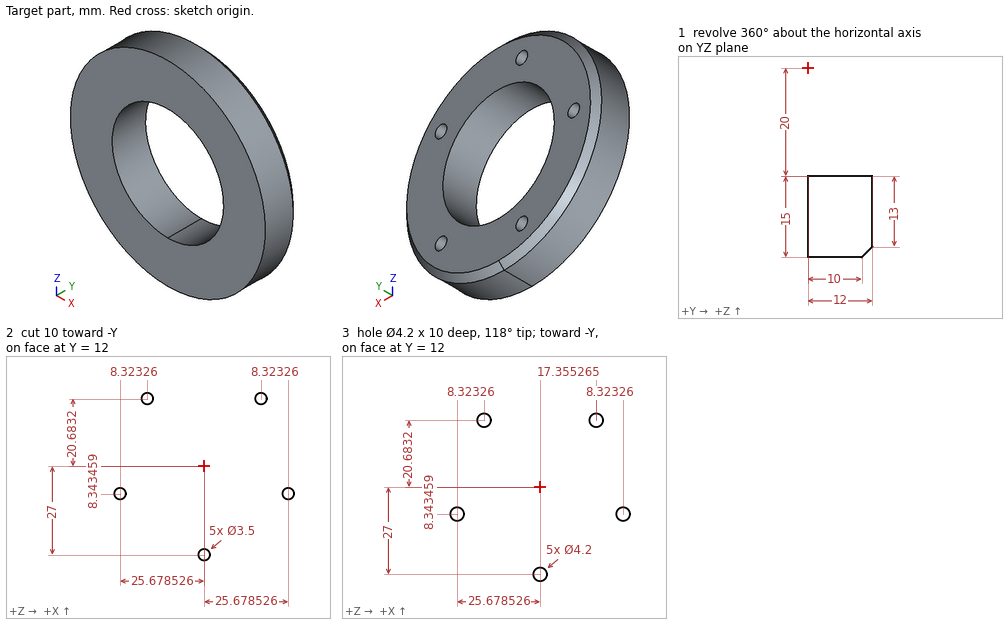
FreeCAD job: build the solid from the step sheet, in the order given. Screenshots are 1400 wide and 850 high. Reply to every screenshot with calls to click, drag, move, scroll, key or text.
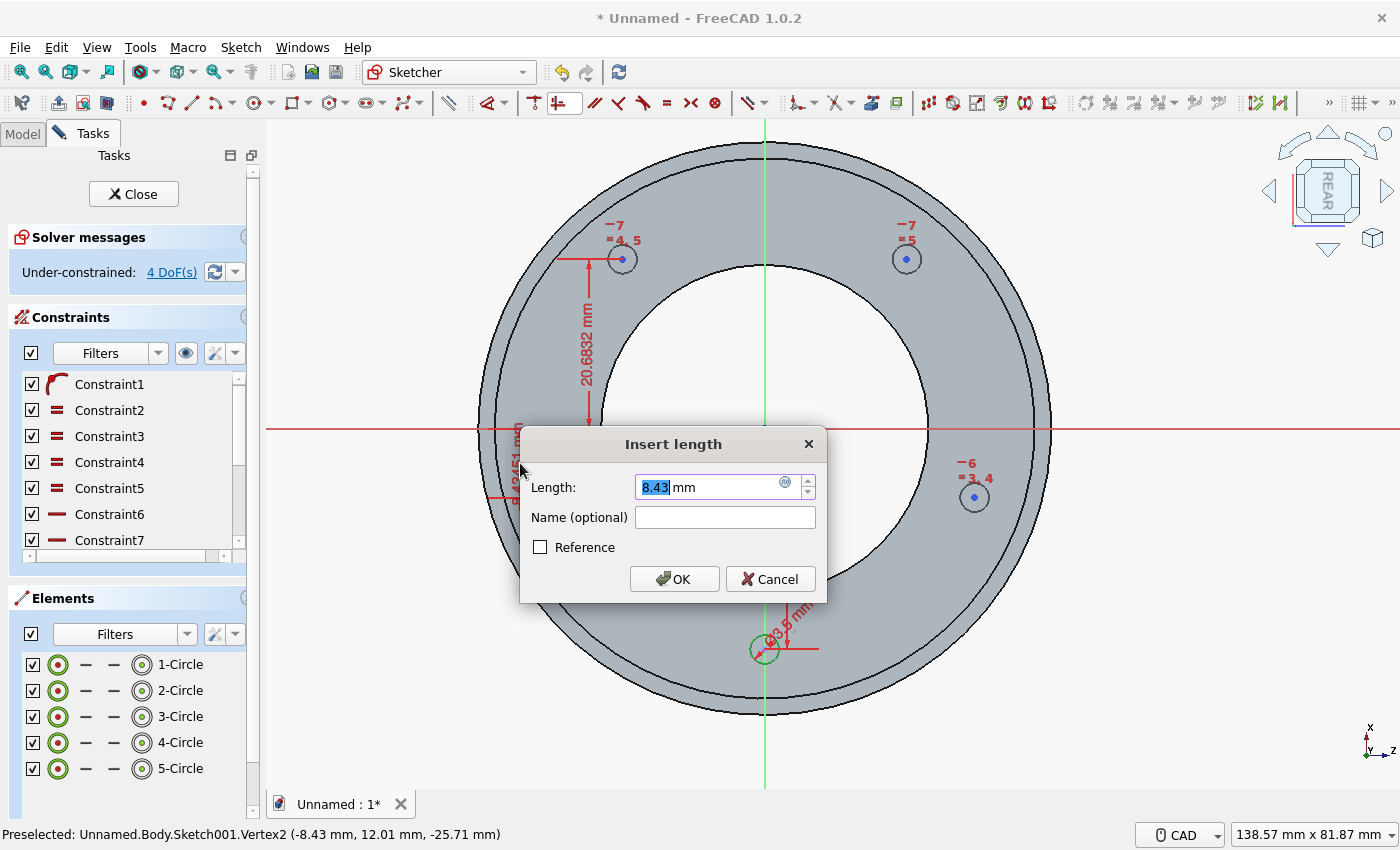
text(8.343459)
key(Return)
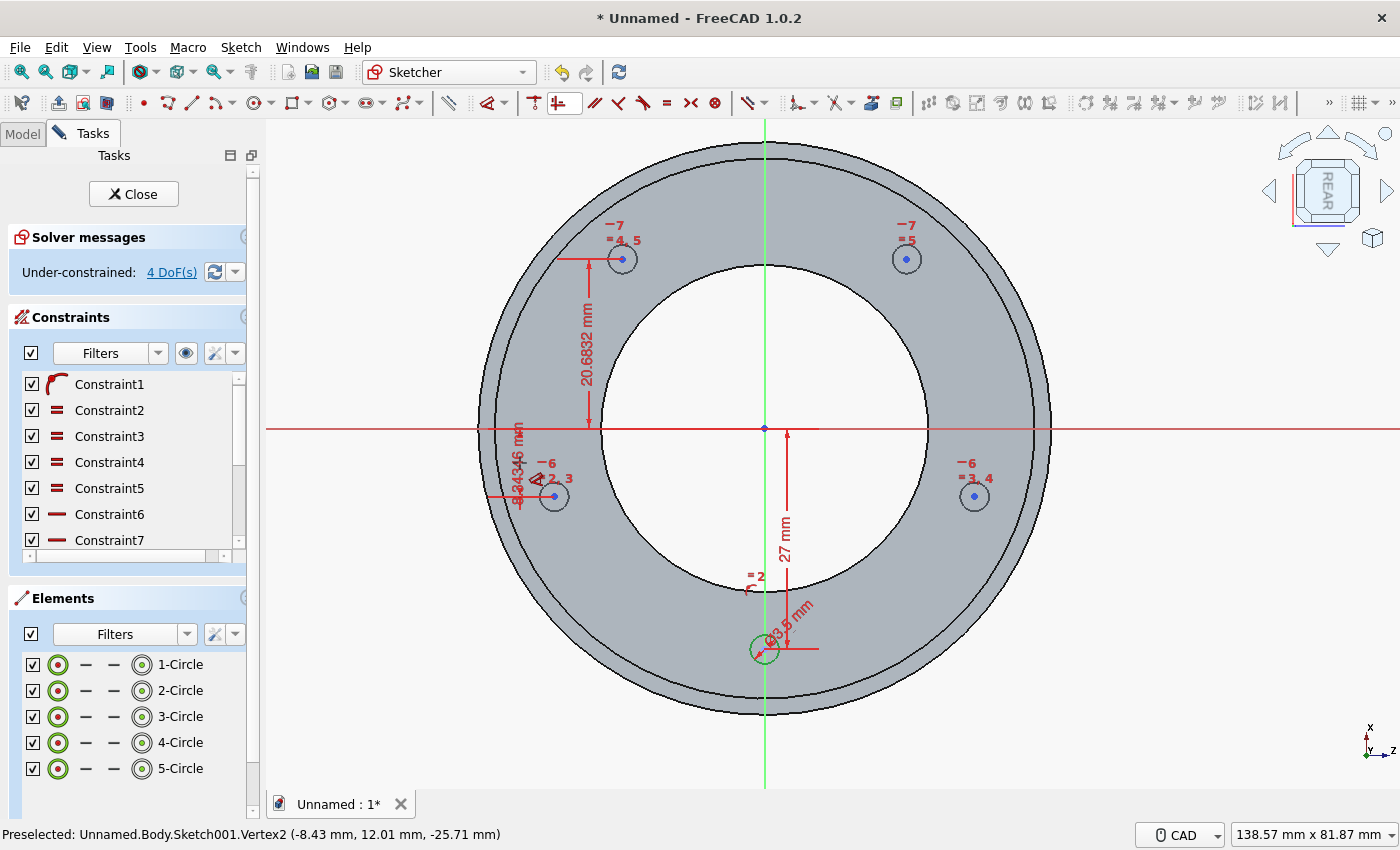
click(554, 497)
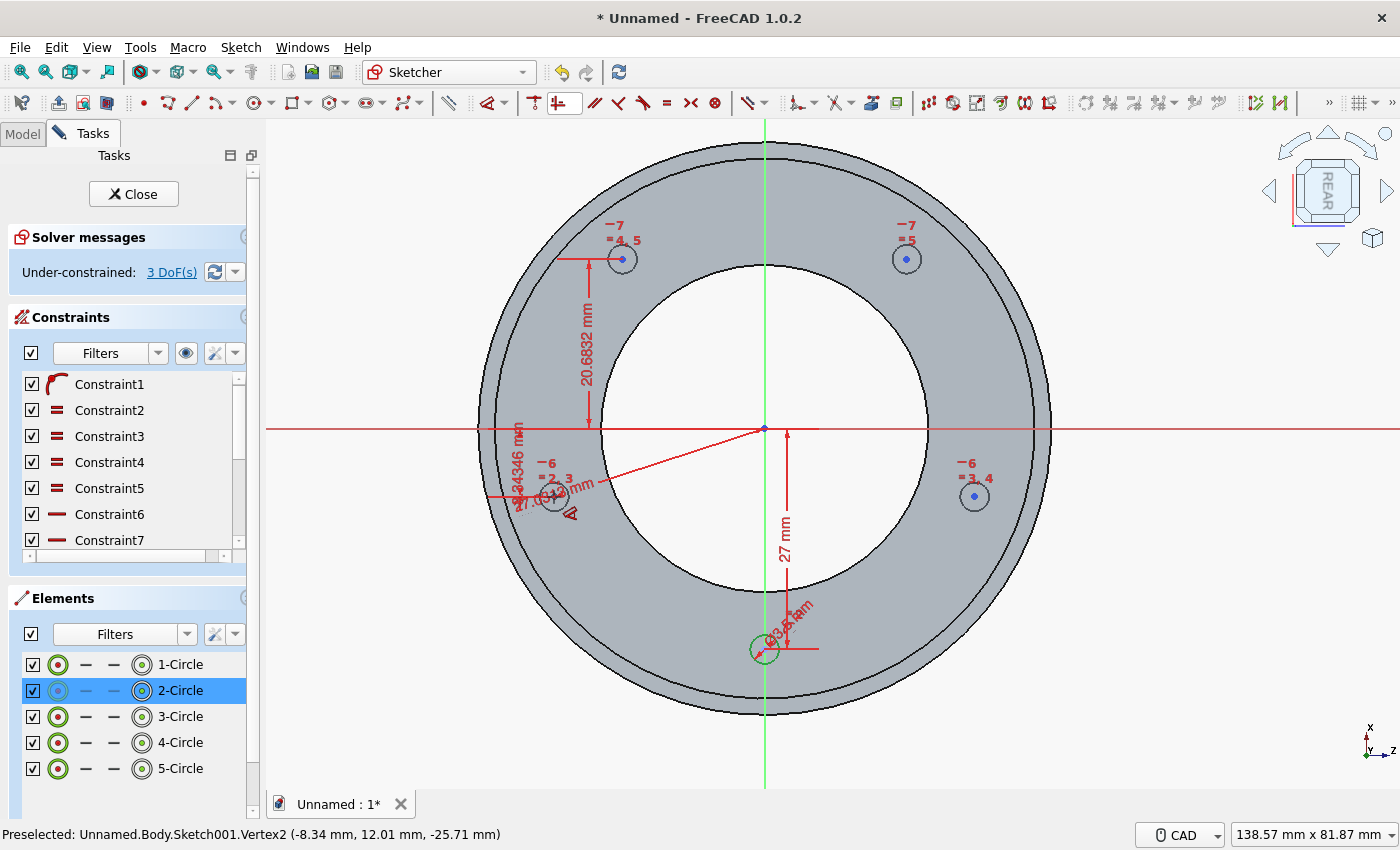
click(623, 259)
click(588, 225)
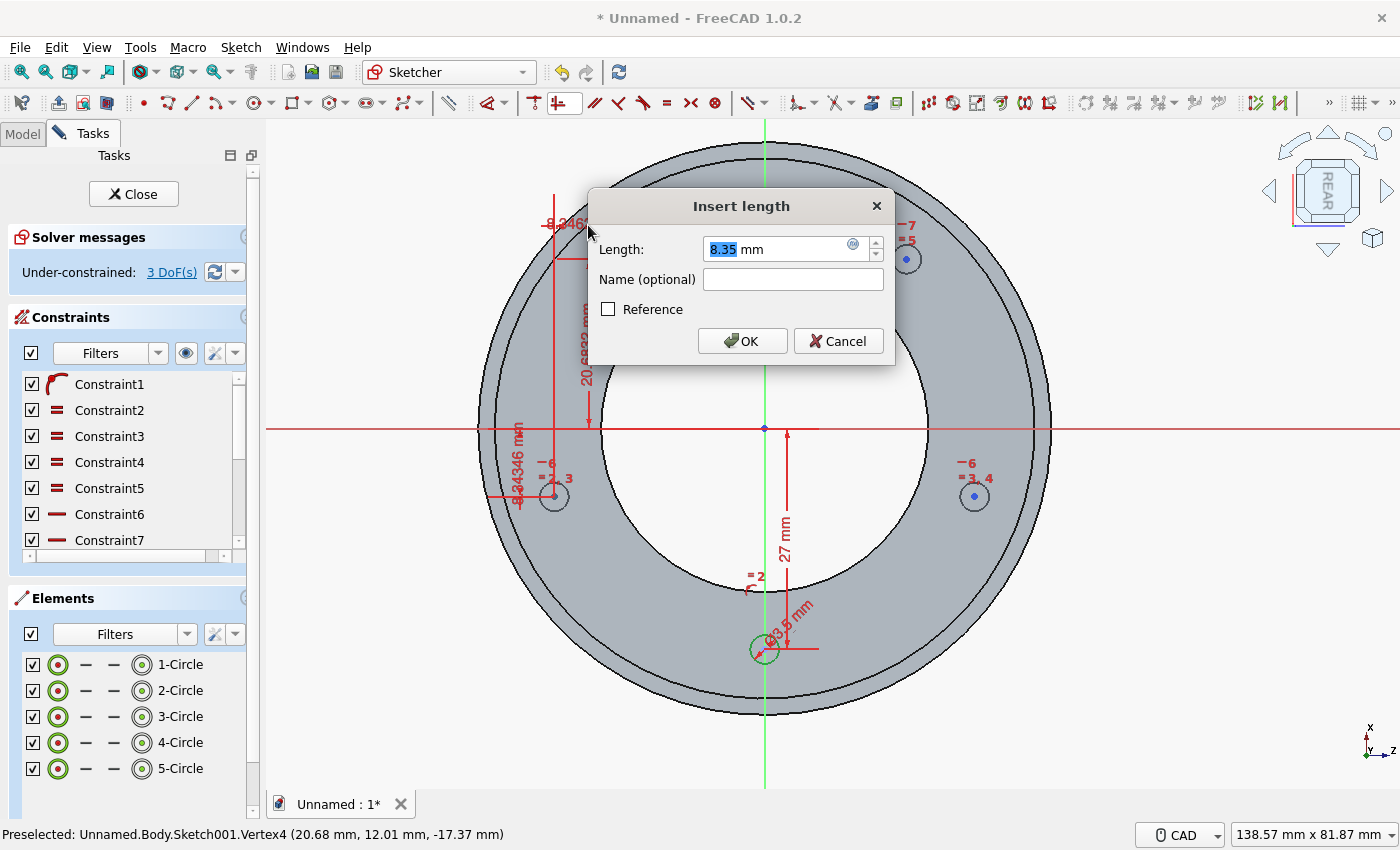
text(8.32326)
key(Return)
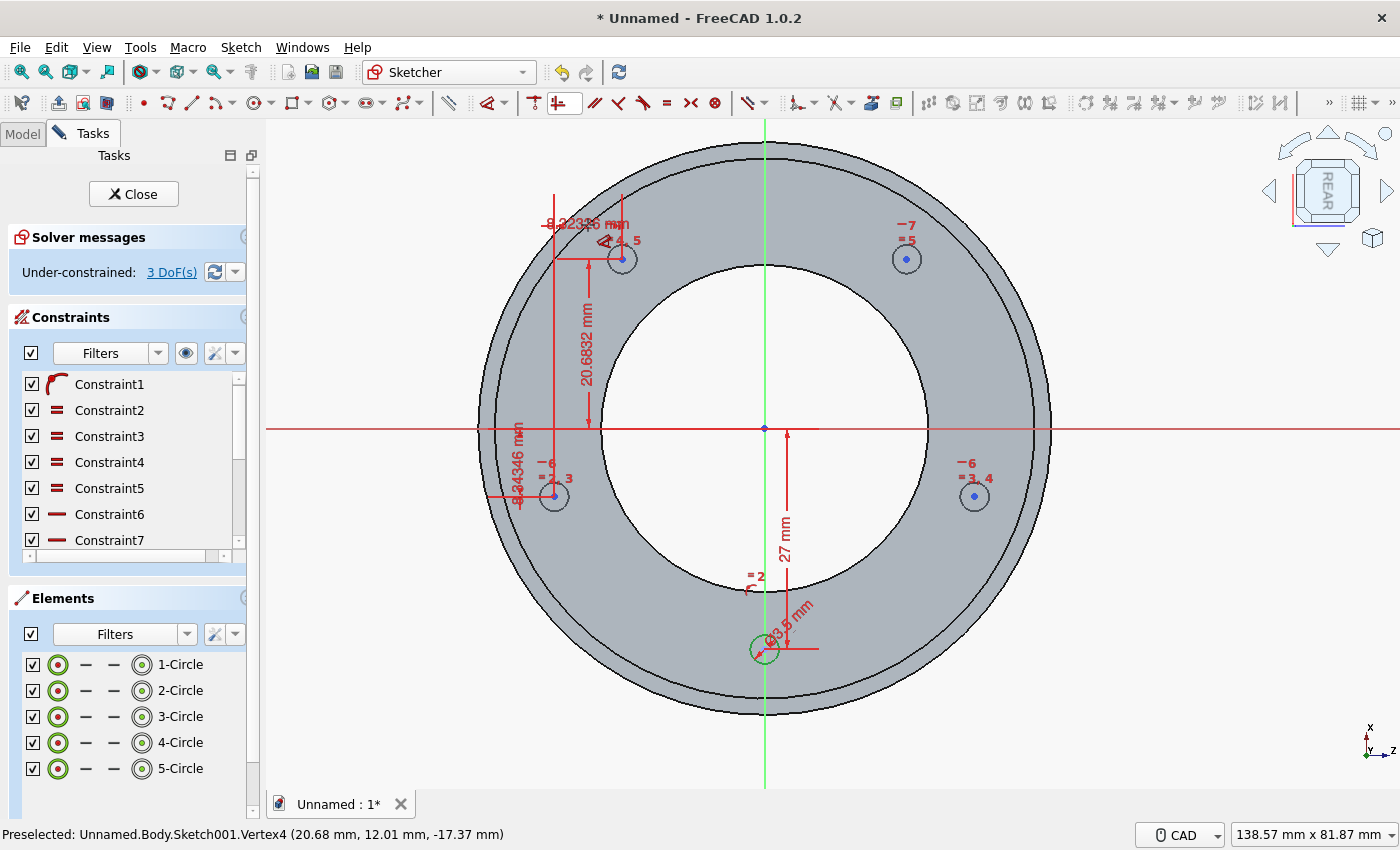
click(975, 497)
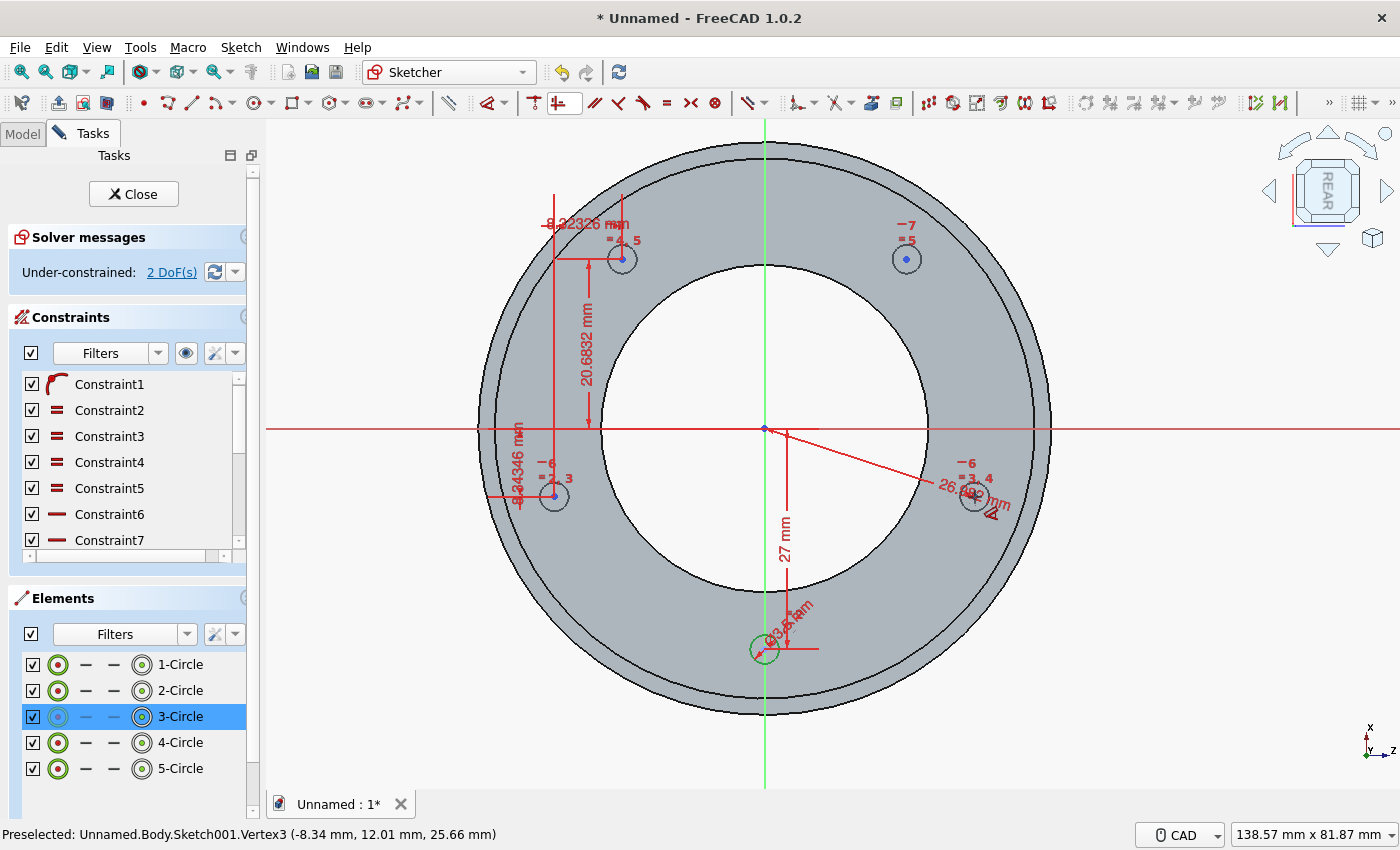
click(907, 259)
click(941, 225)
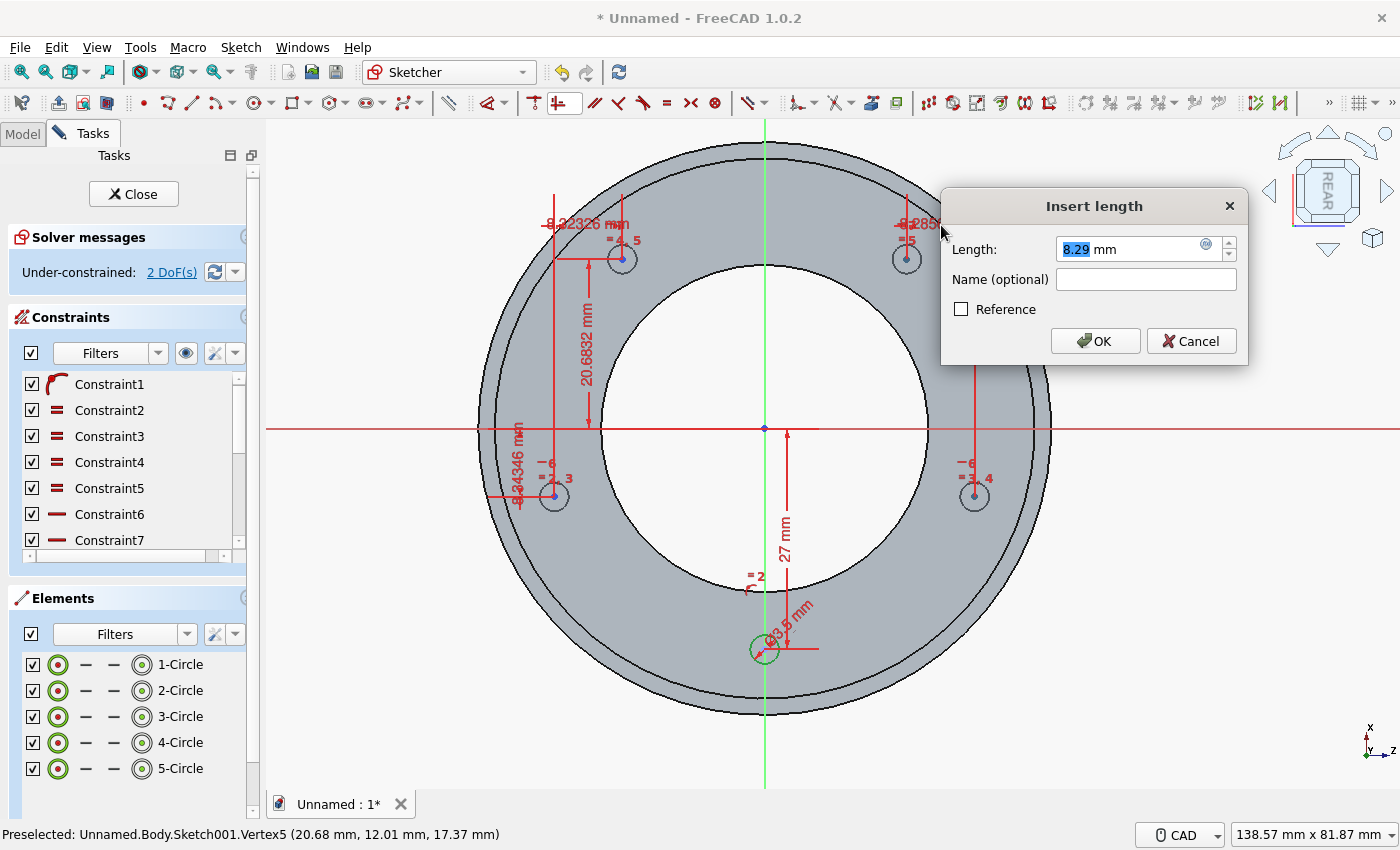
text(8.32326)
key(Return)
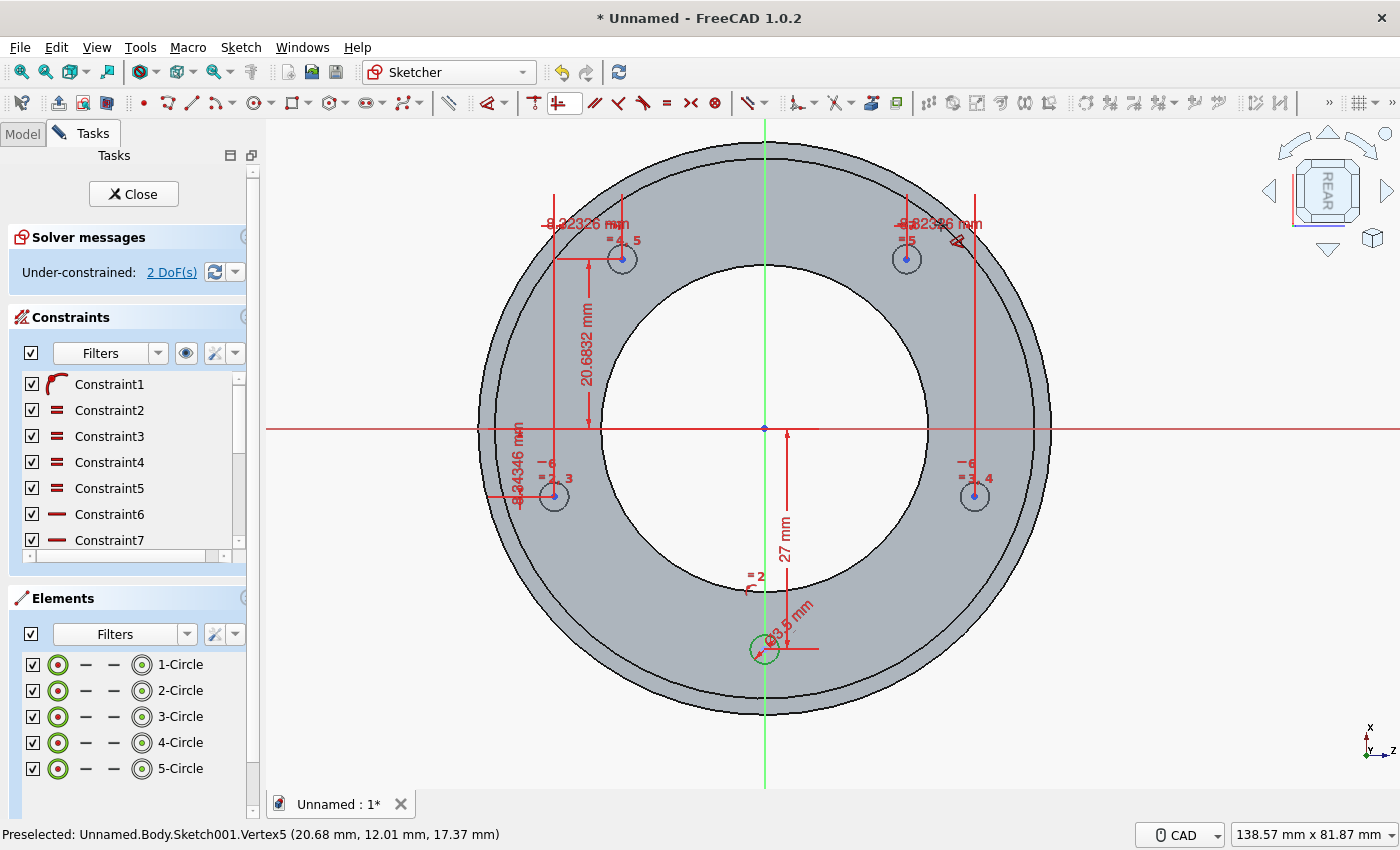
click(554, 497)
click(659, 531)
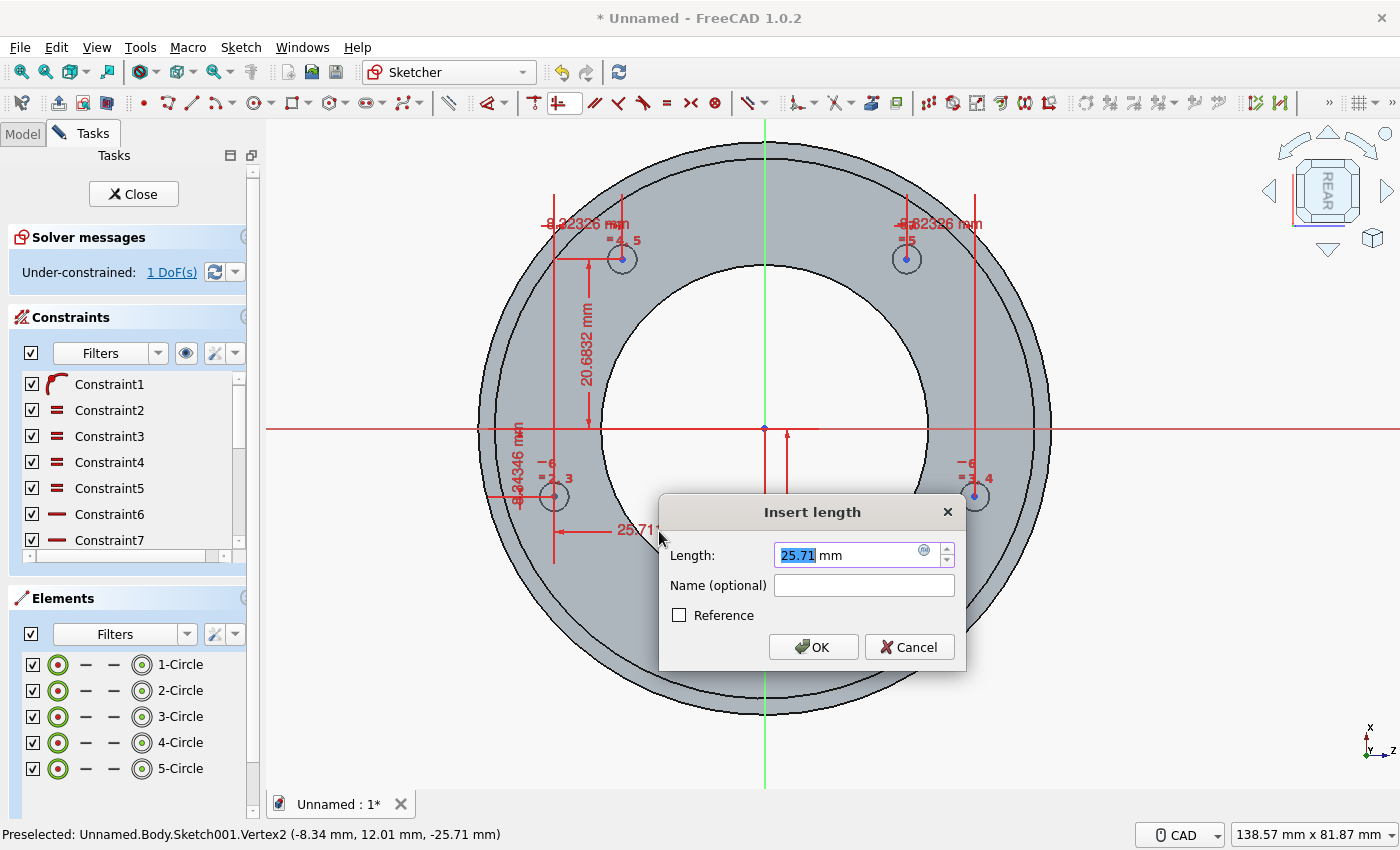
text(25.678526)
key(Return)